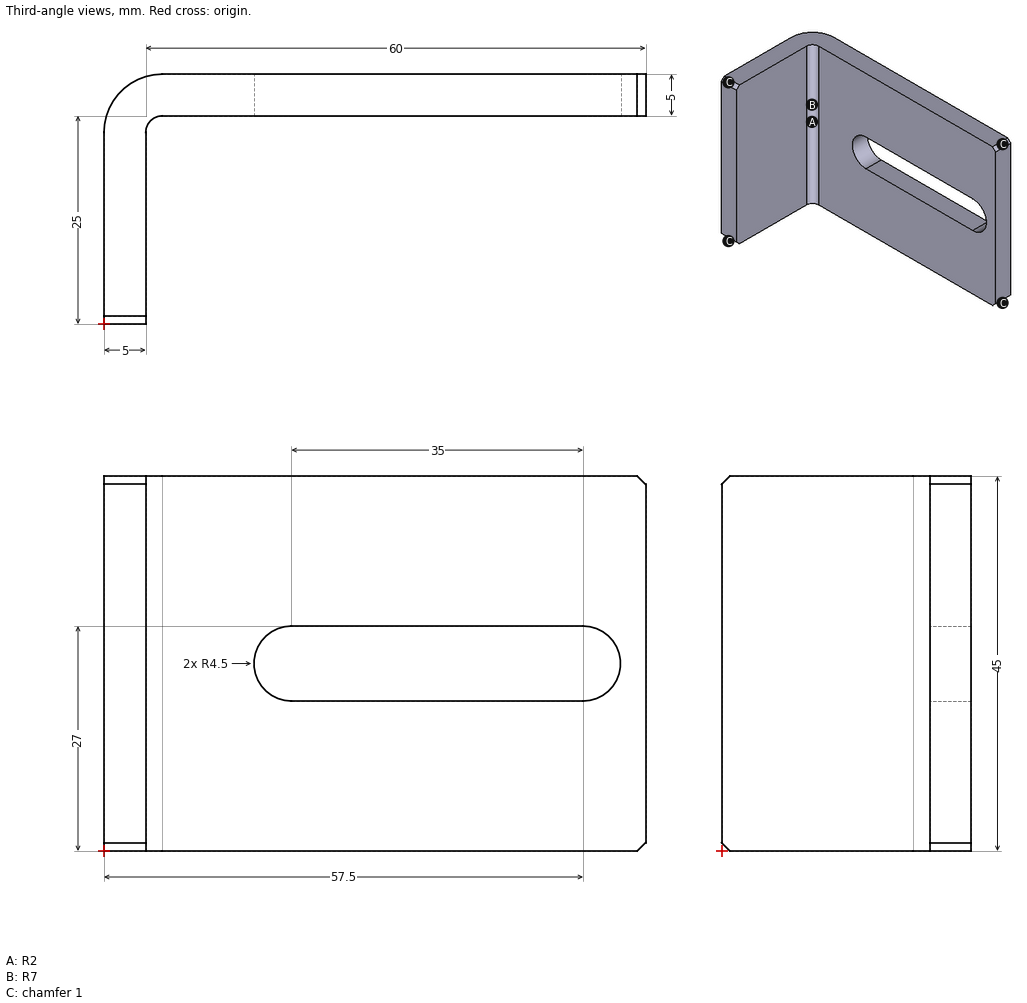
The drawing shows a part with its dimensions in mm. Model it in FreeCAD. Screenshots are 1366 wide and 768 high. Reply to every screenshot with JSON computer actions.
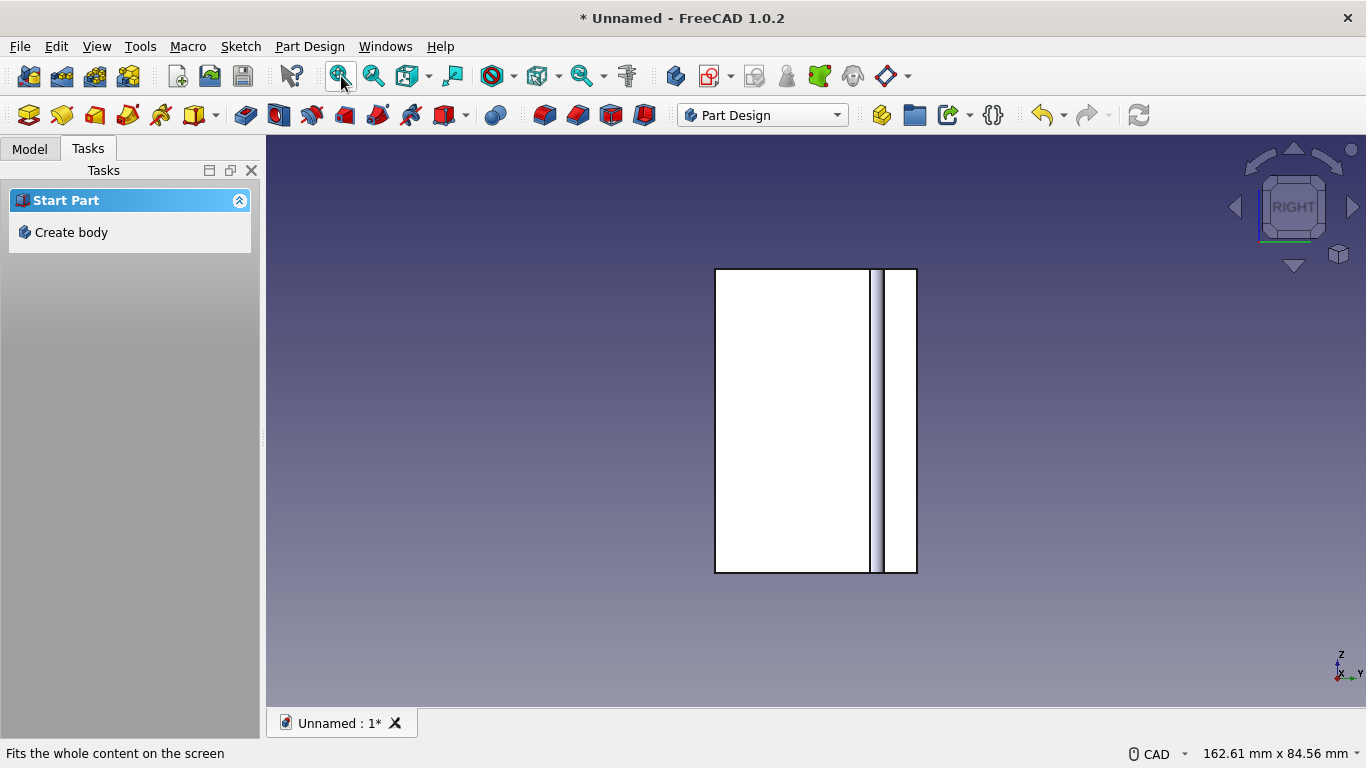
{"action": "key", "text": "5"}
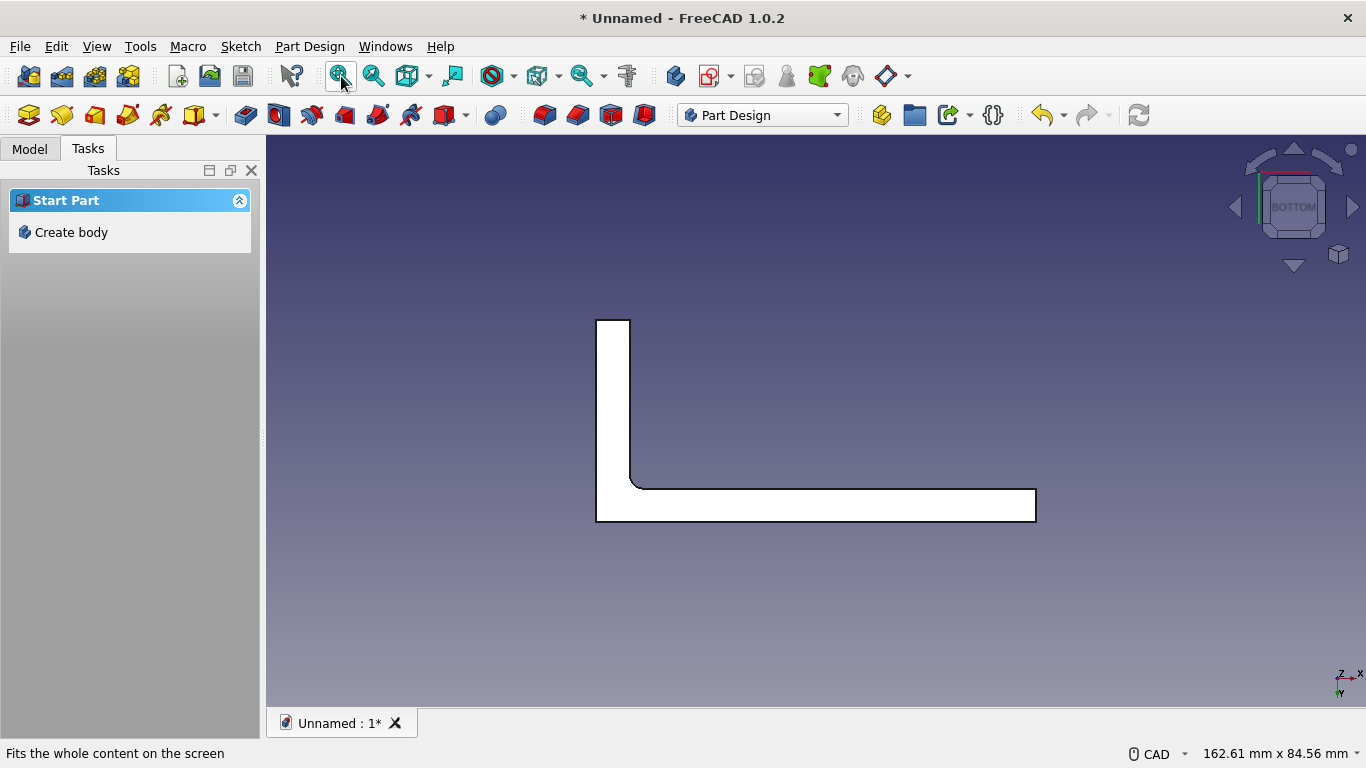
{"action": "left_click", "coordinate": [341, 76]}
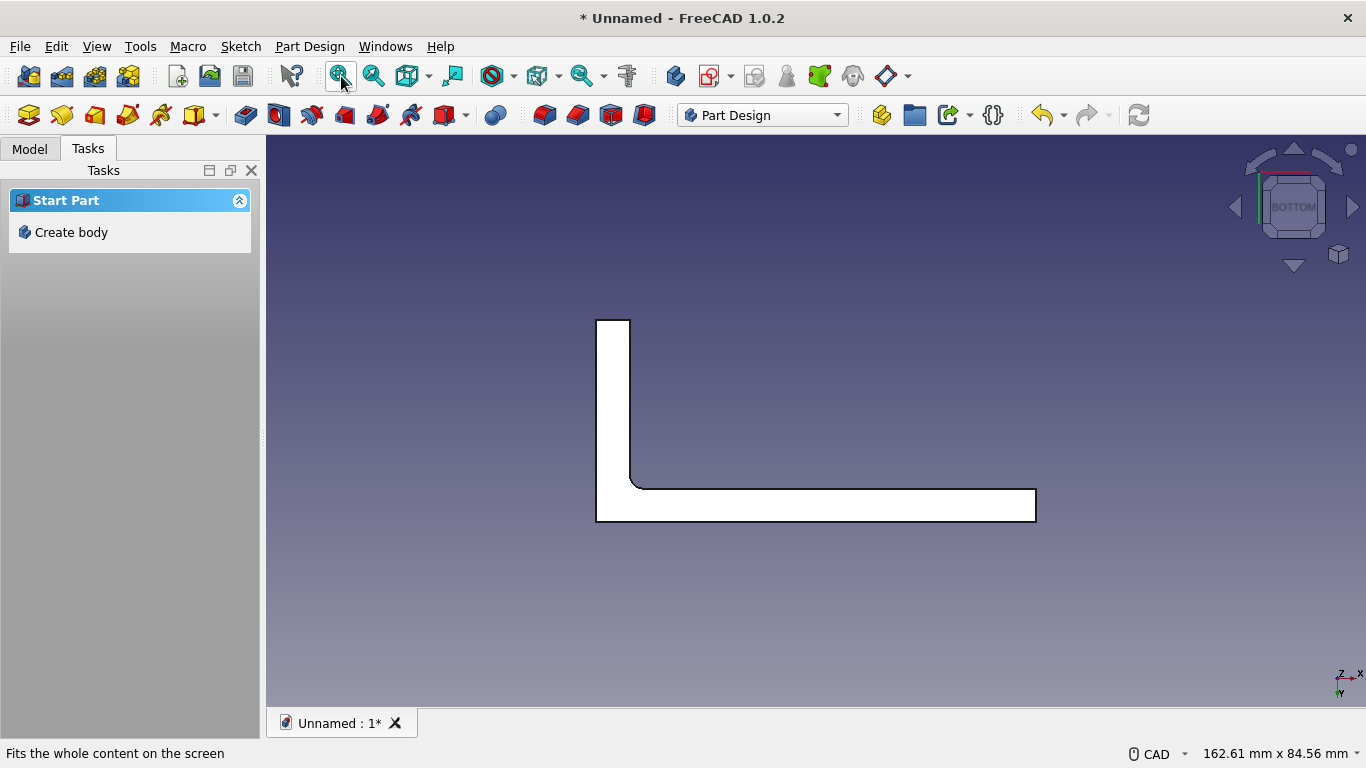
{"action": "key", "text": "4"}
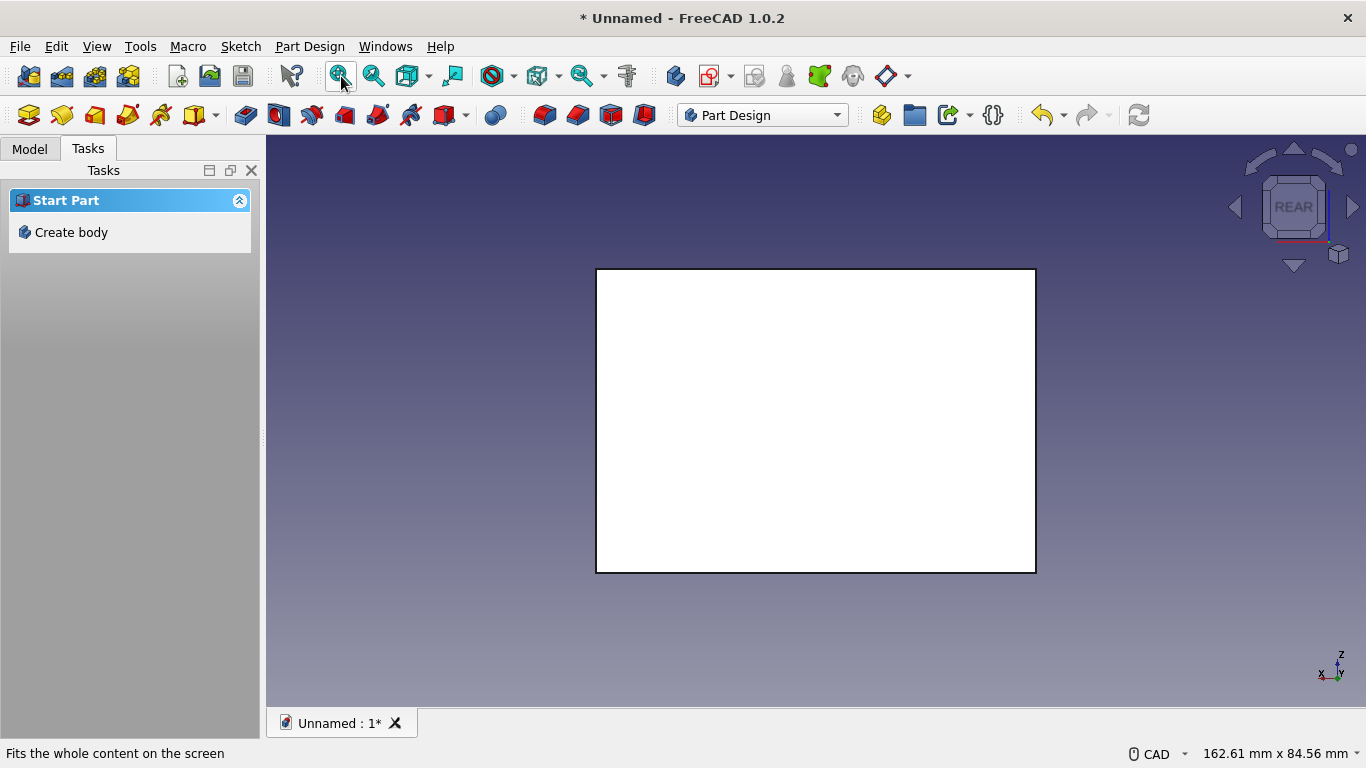
{"action": "left_click", "coordinate": [1036, 420]}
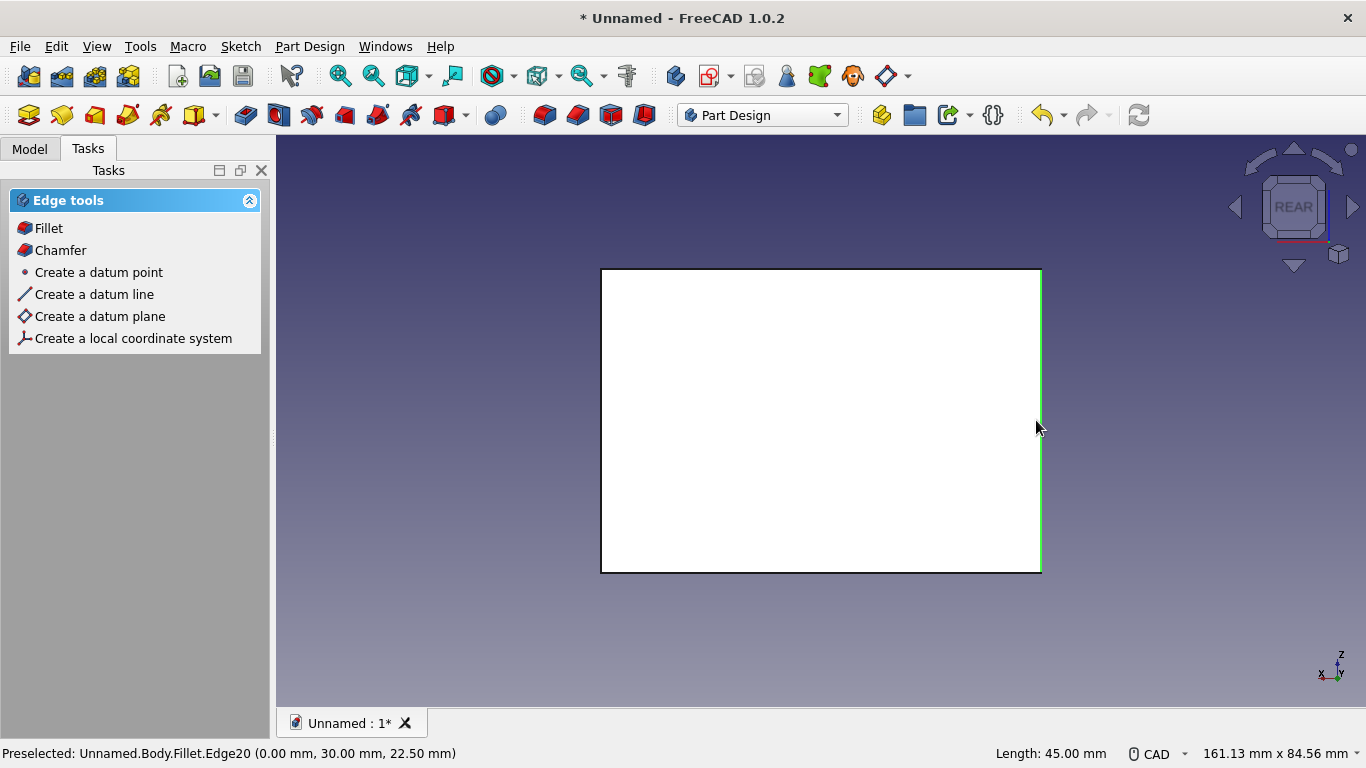
{"action": "left_click", "coordinate": [545, 116]}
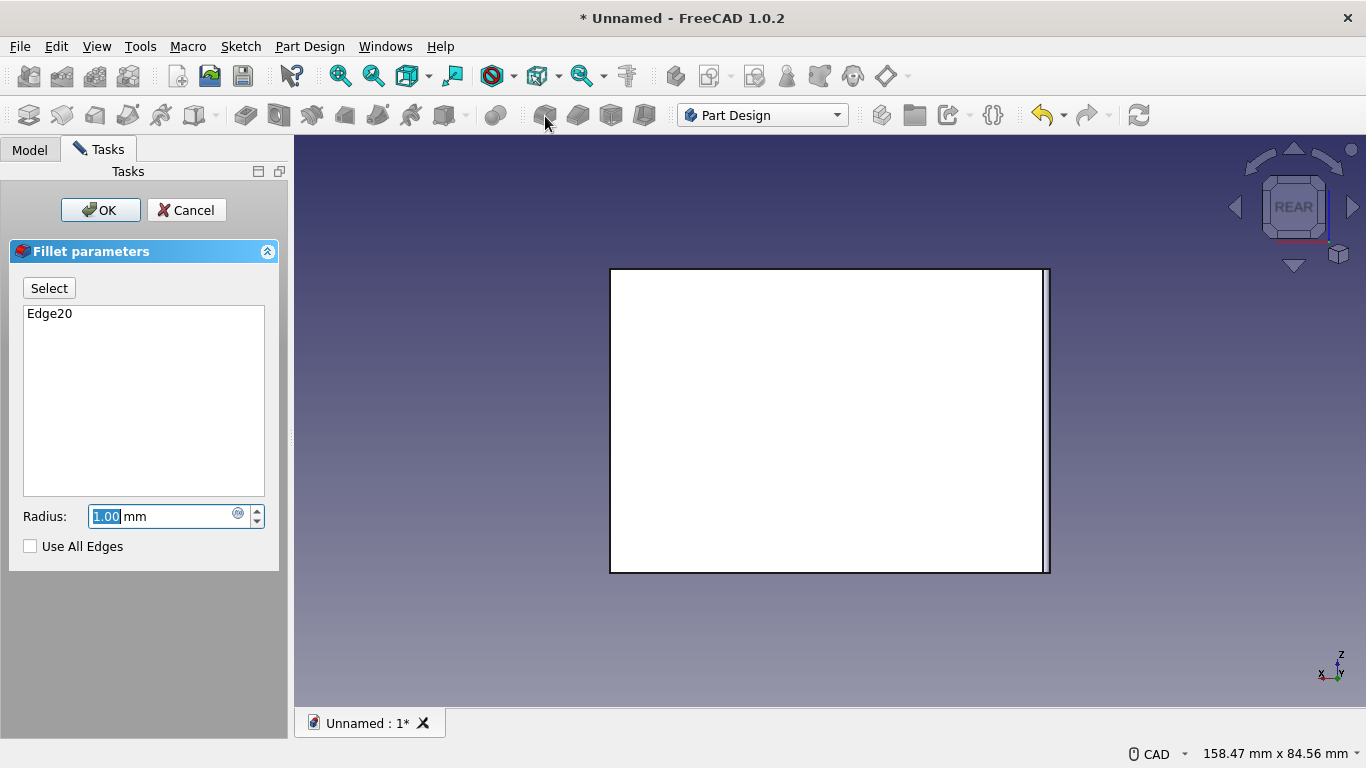
{"action": "type", "text": "7"}
{"action": "key", "text": "Tab"}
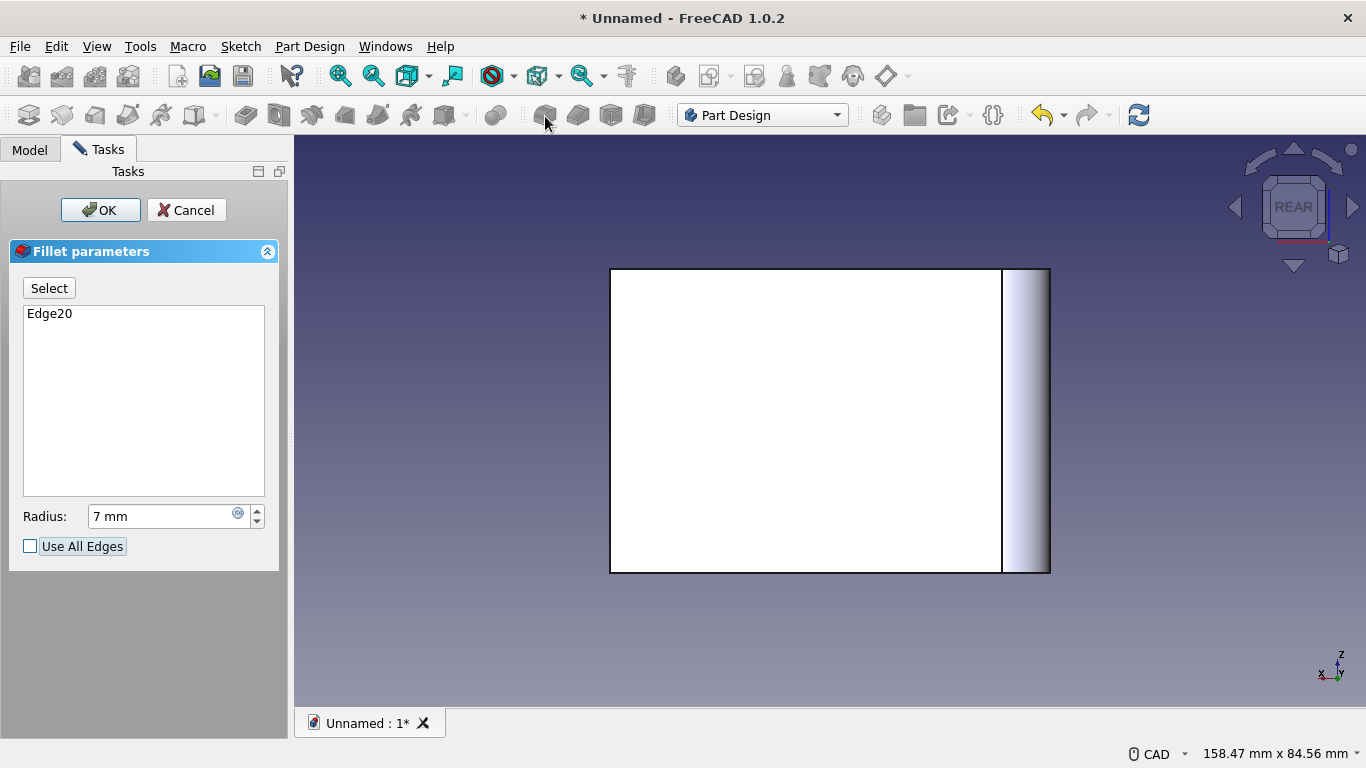
{"action": "left_click", "coordinate": [101, 210]}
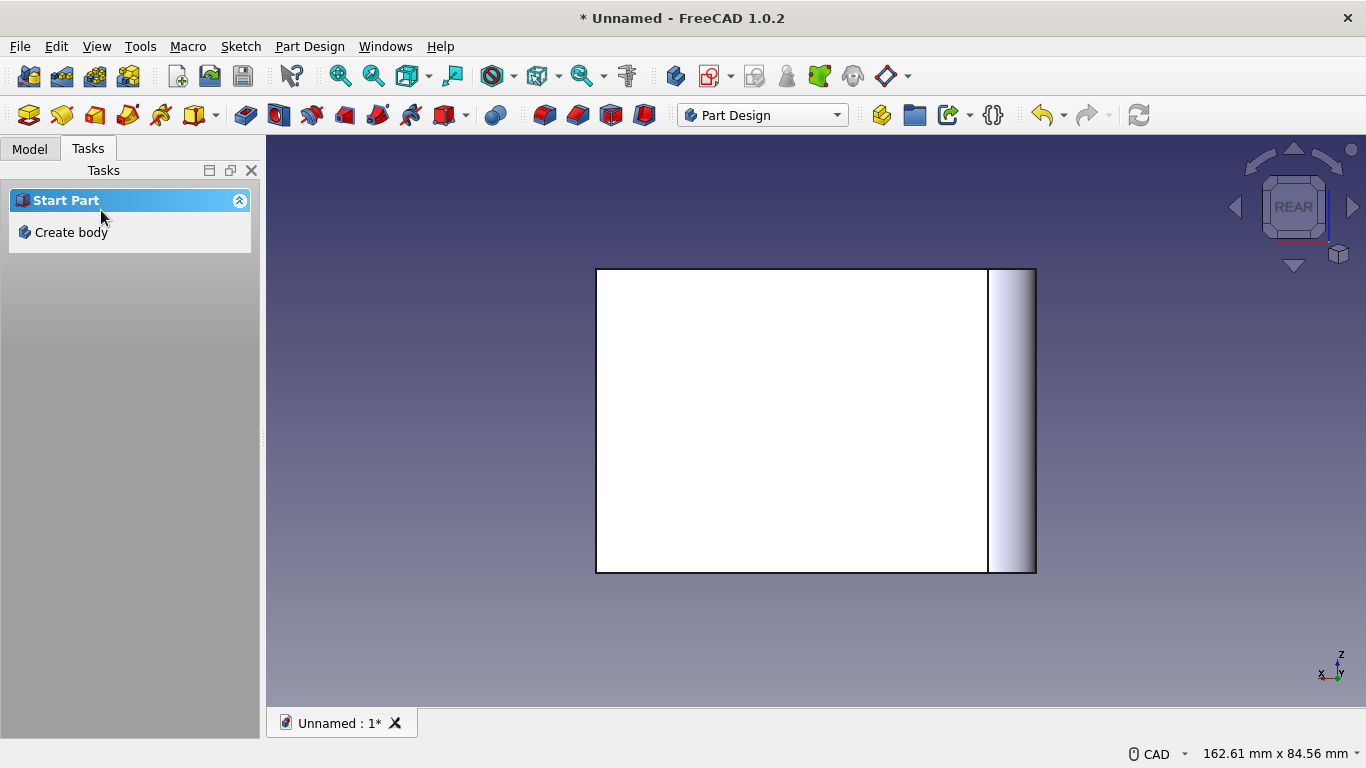
{"action": "key", "text": "0"}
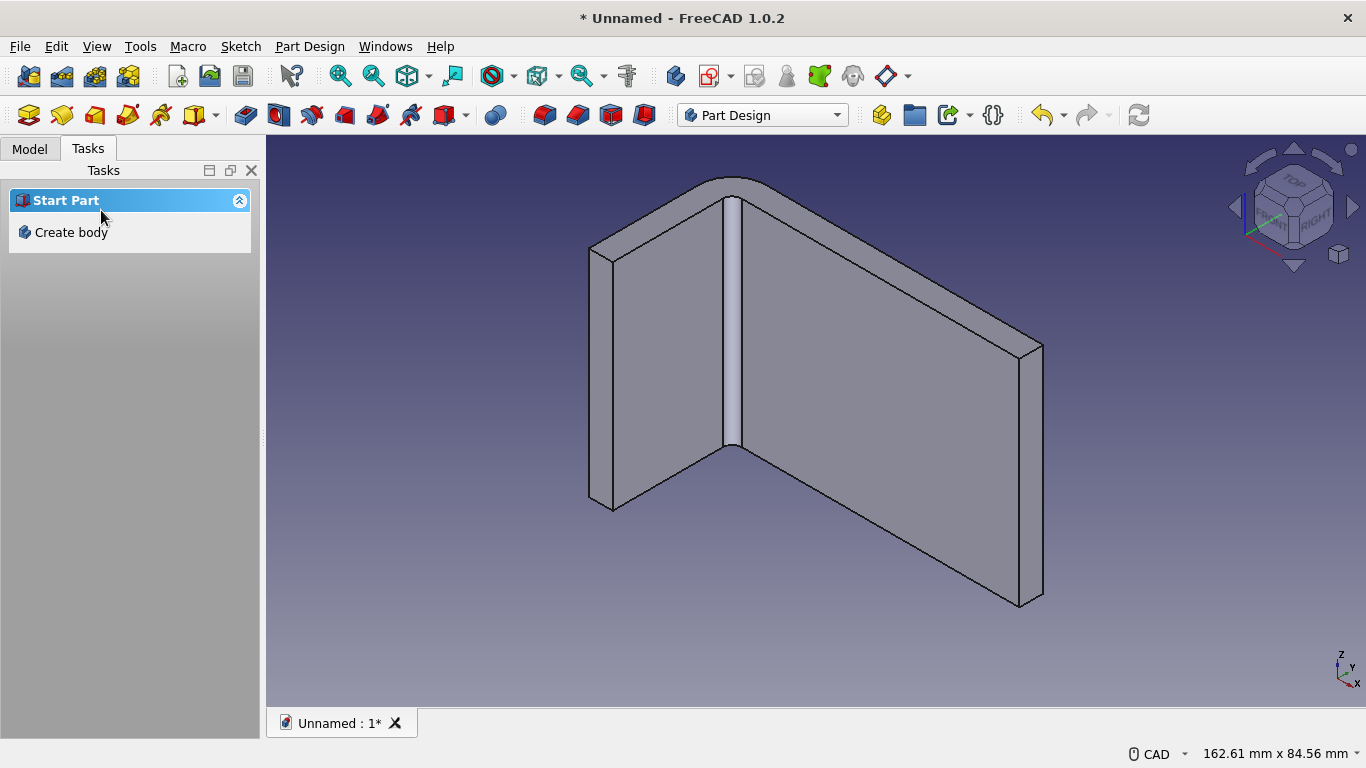
{"action": "left_click", "coordinate": [601, 254]}